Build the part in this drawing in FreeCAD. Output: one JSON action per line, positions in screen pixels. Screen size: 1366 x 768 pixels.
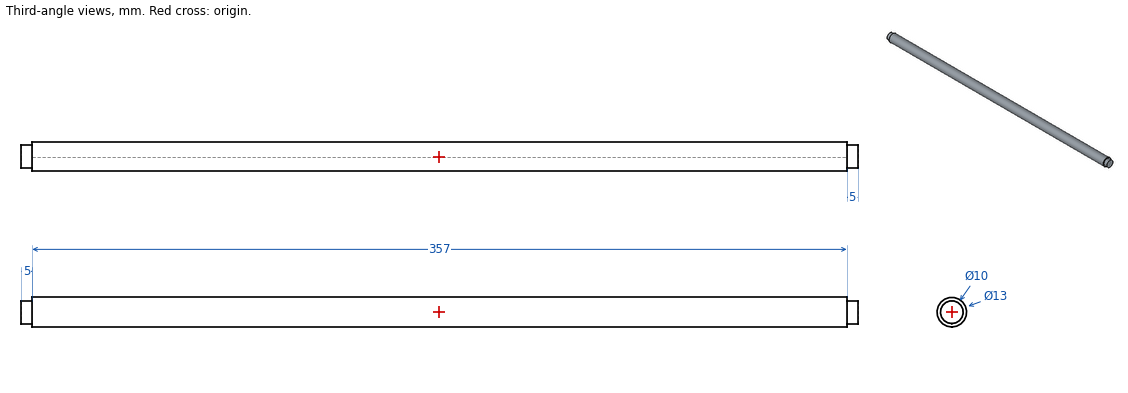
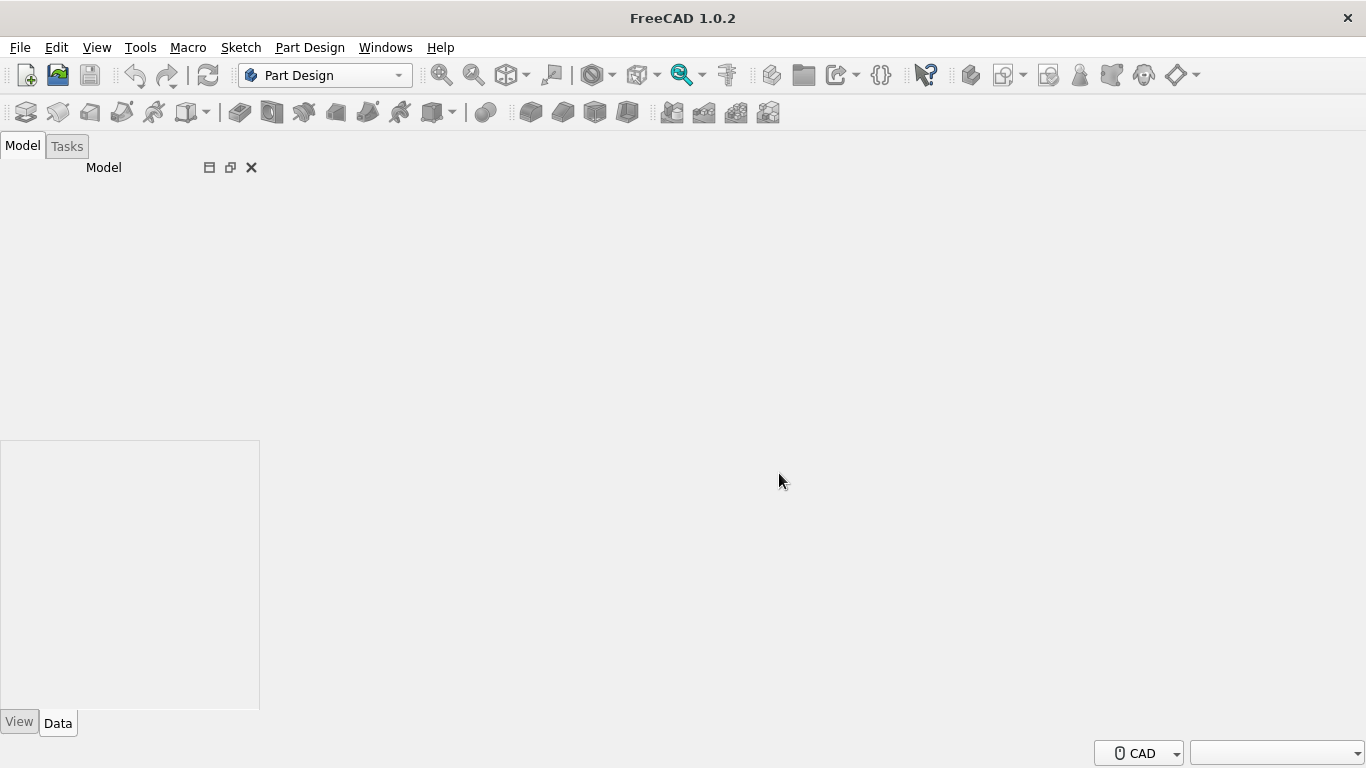
{"action": "left_click", "coordinate": [26, 76]}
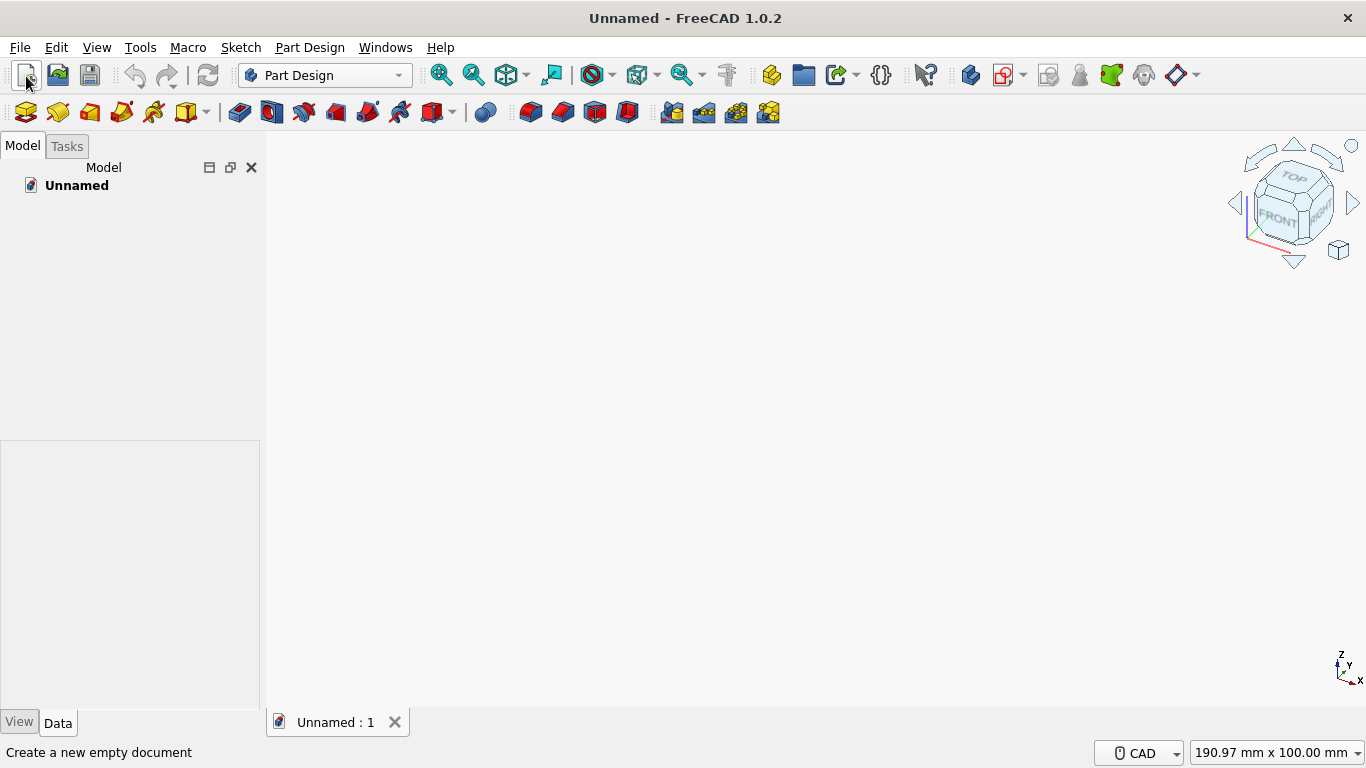
{"action": "left_click", "coordinate": [1004, 76]}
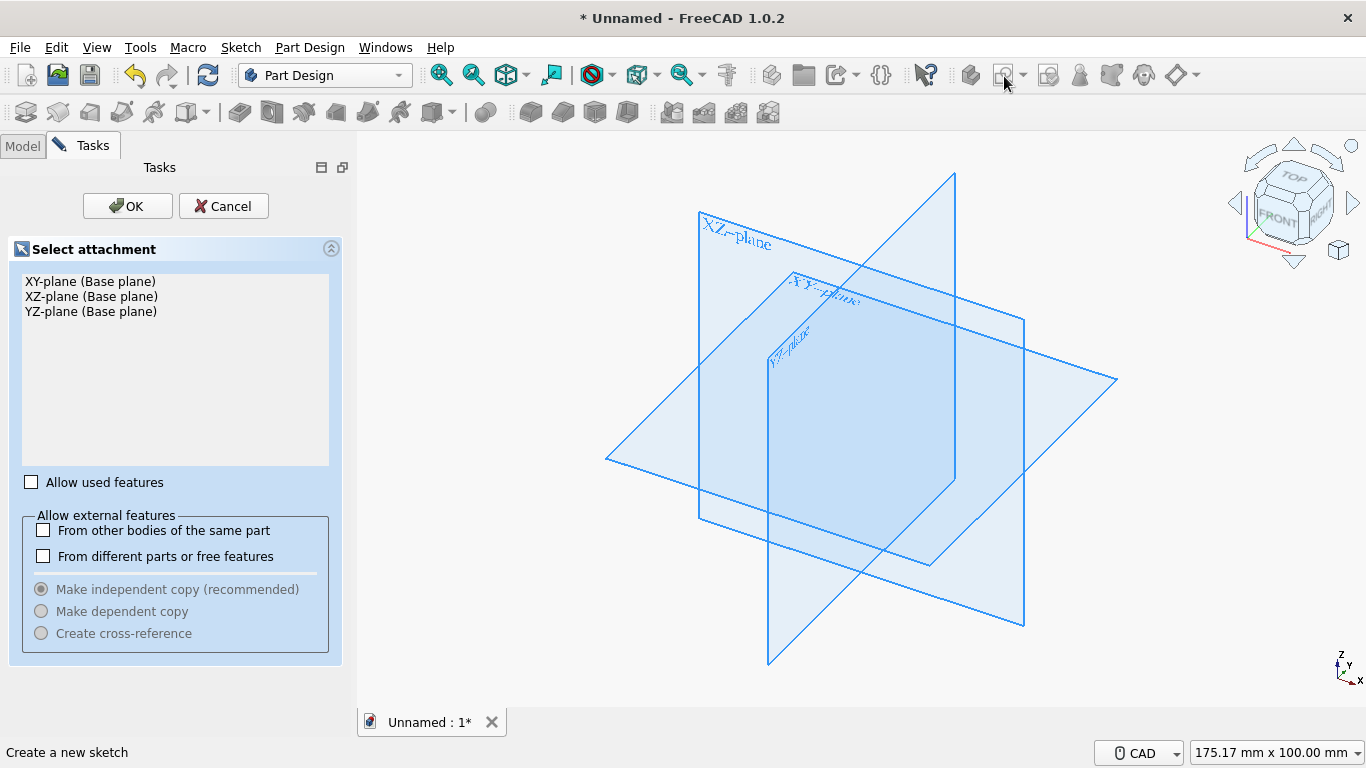
{"action": "left_click", "coordinate": [82, 312]}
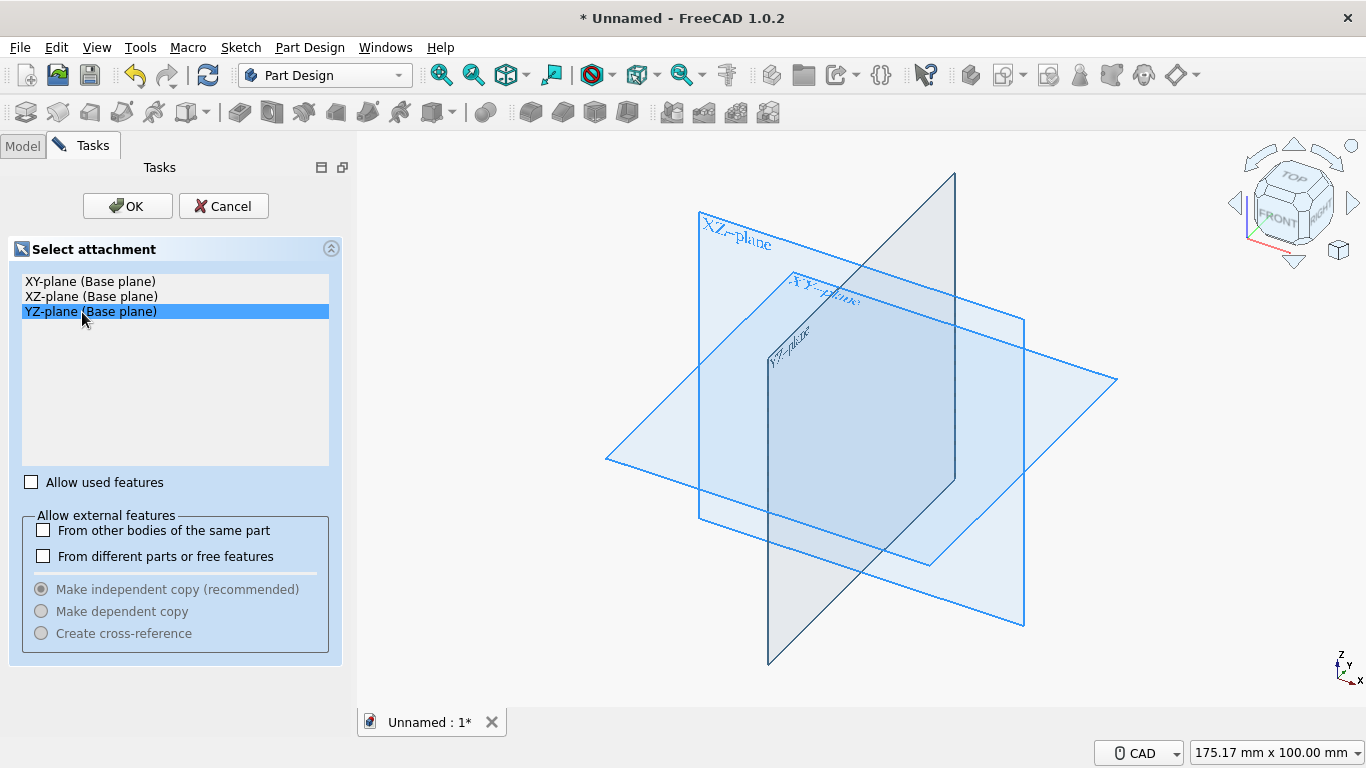
{"action": "left_click", "coordinate": [128, 206]}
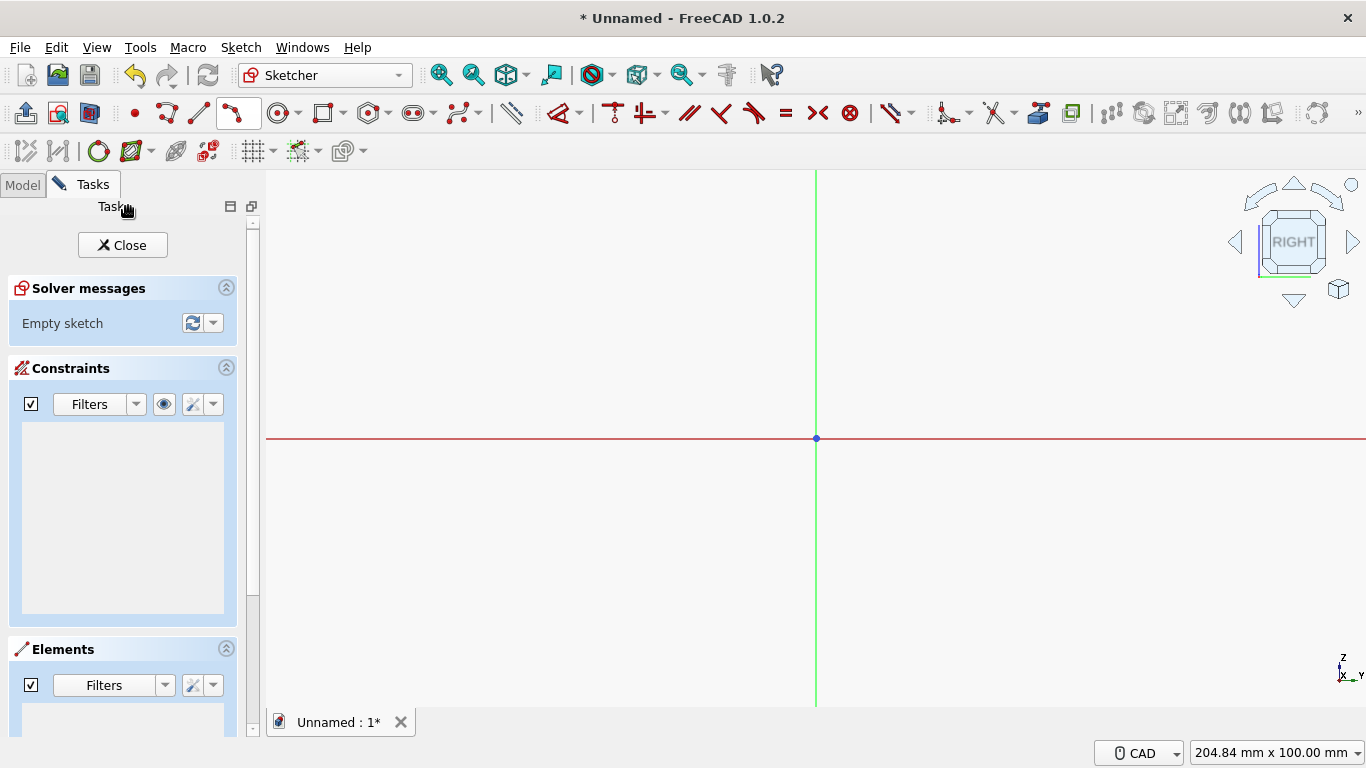
{"action": "scroll", "coordinate": [833, 438], "scroll_direction": "up", "scroll_amount": 8}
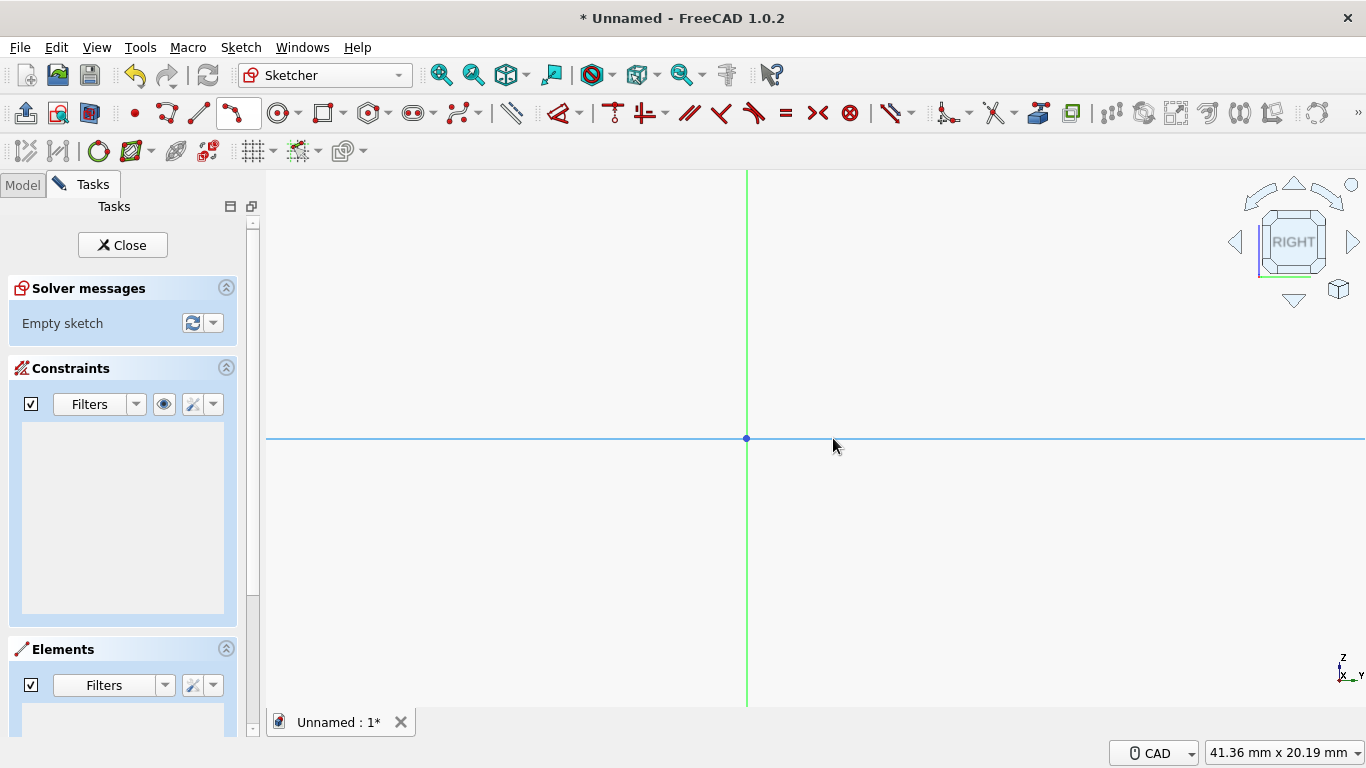
{"action": "left_click", "coordinate": [278, 114]}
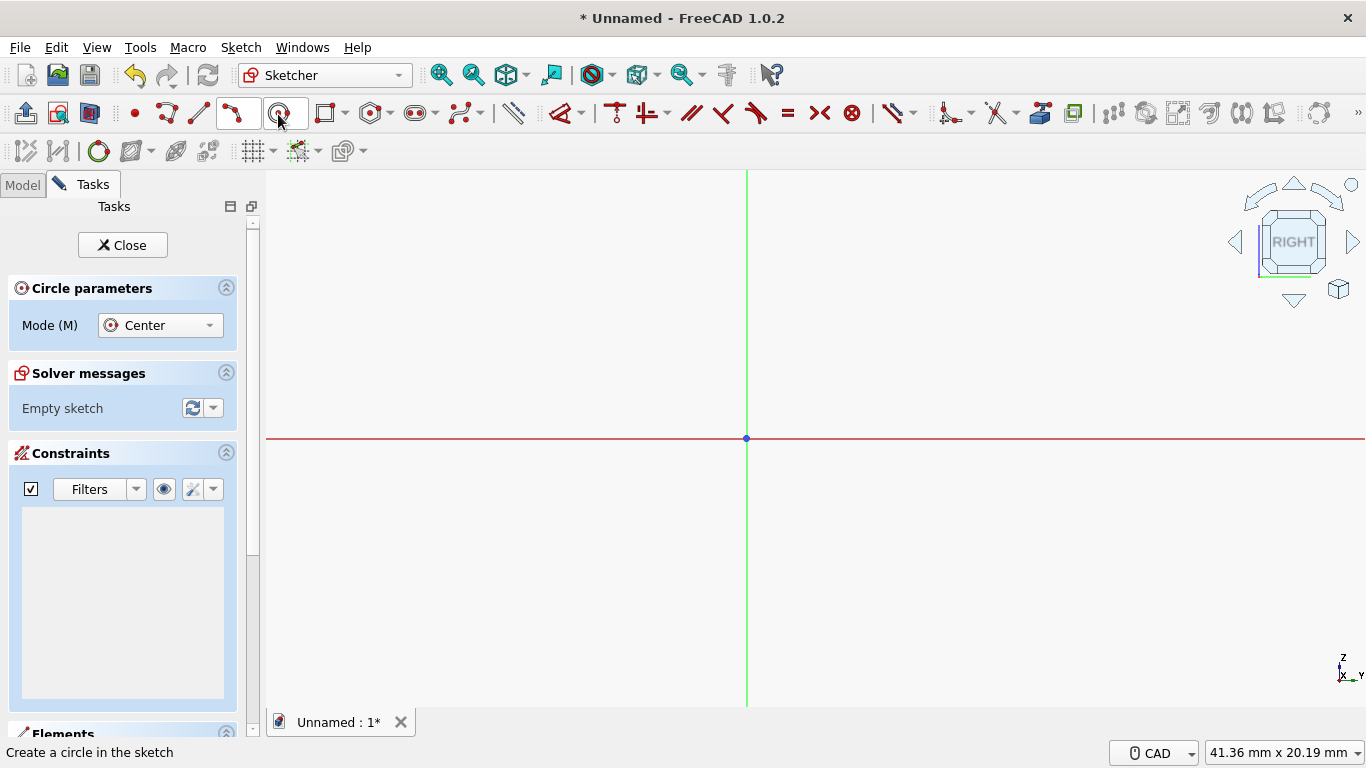
{"action": "left_click", "coordinate": [747, 438]}
{"action": "left_click", "coordinate": [869, 316]}
{"action": "key", "text": "Escape"}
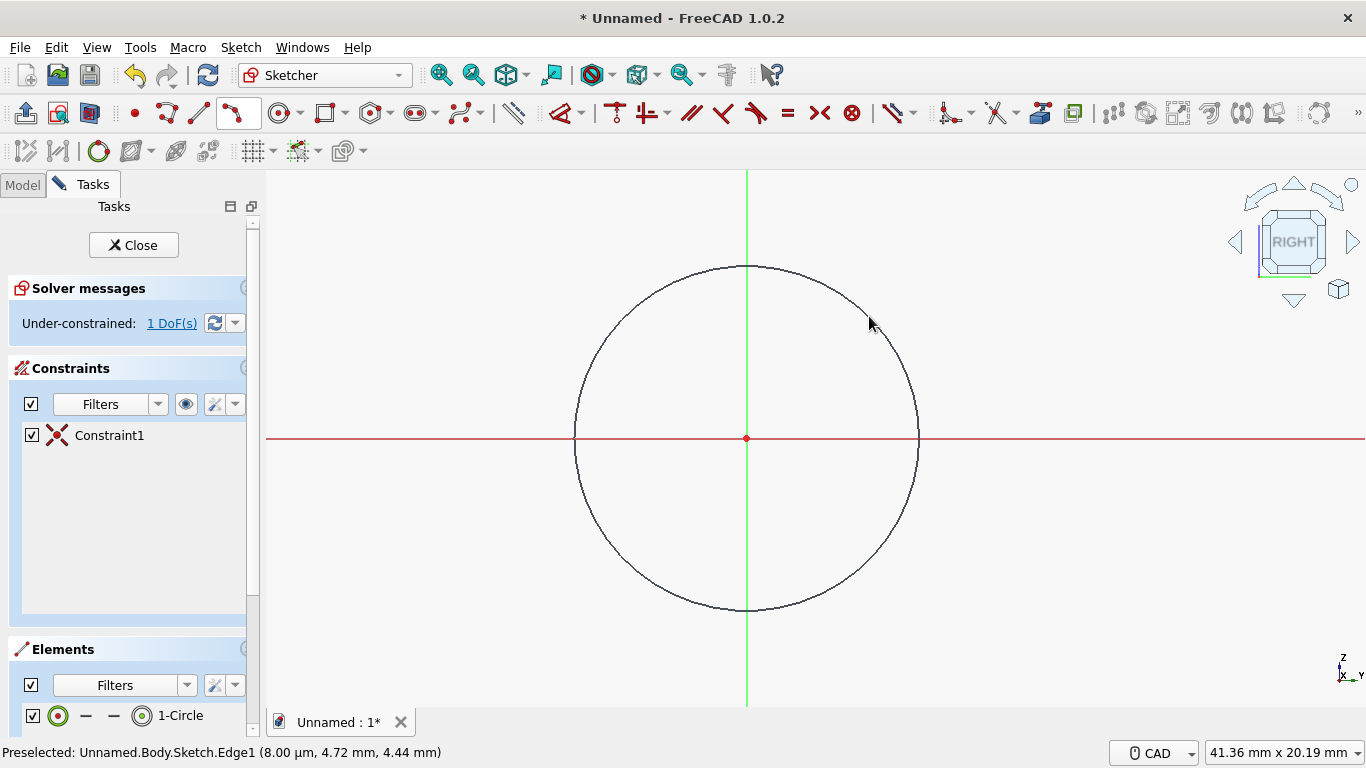
{"action": "left_click", "coordinate": [868, 316]}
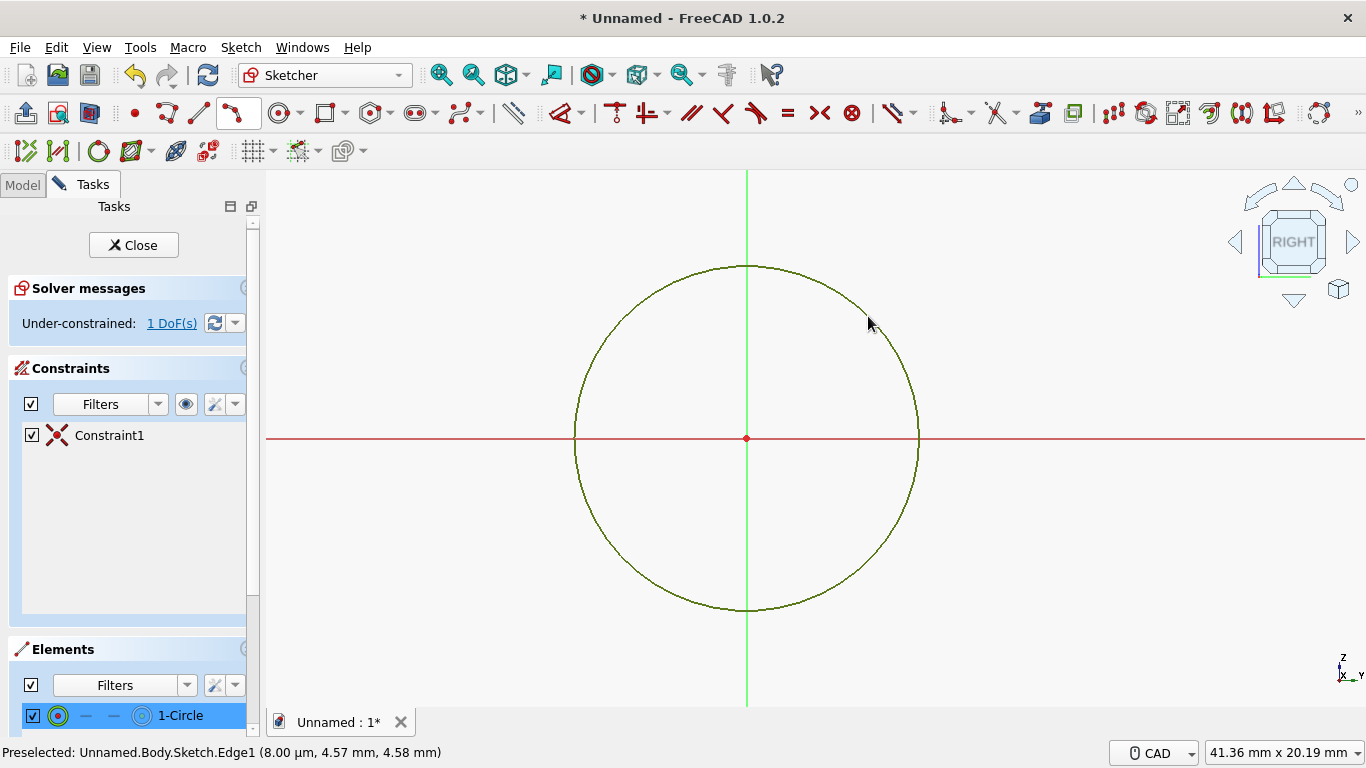
{"action": "key", "text": "k o"}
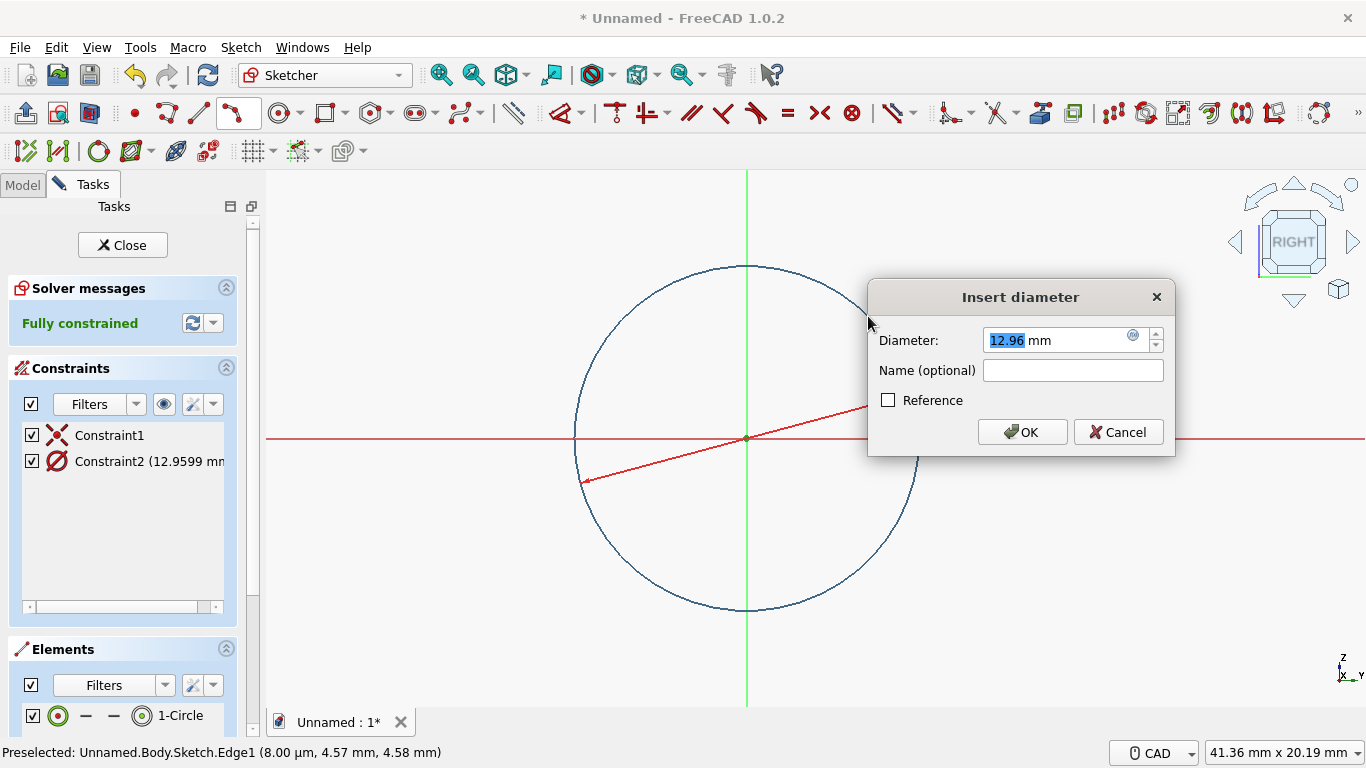
{"action": "type", "text": "13"}
{"action": "key", "text": "Return"}